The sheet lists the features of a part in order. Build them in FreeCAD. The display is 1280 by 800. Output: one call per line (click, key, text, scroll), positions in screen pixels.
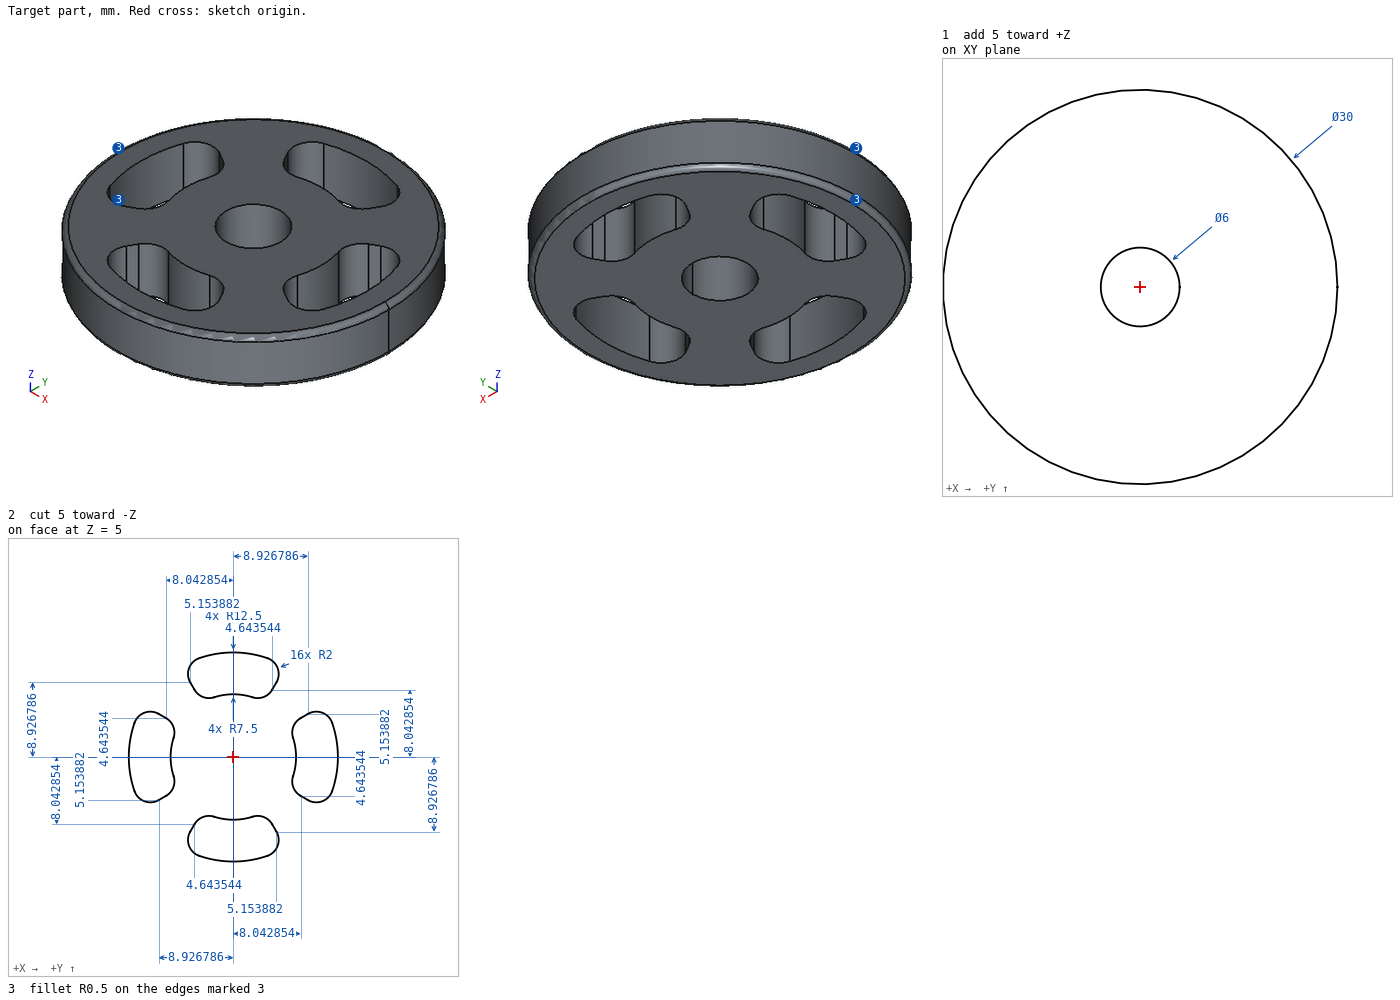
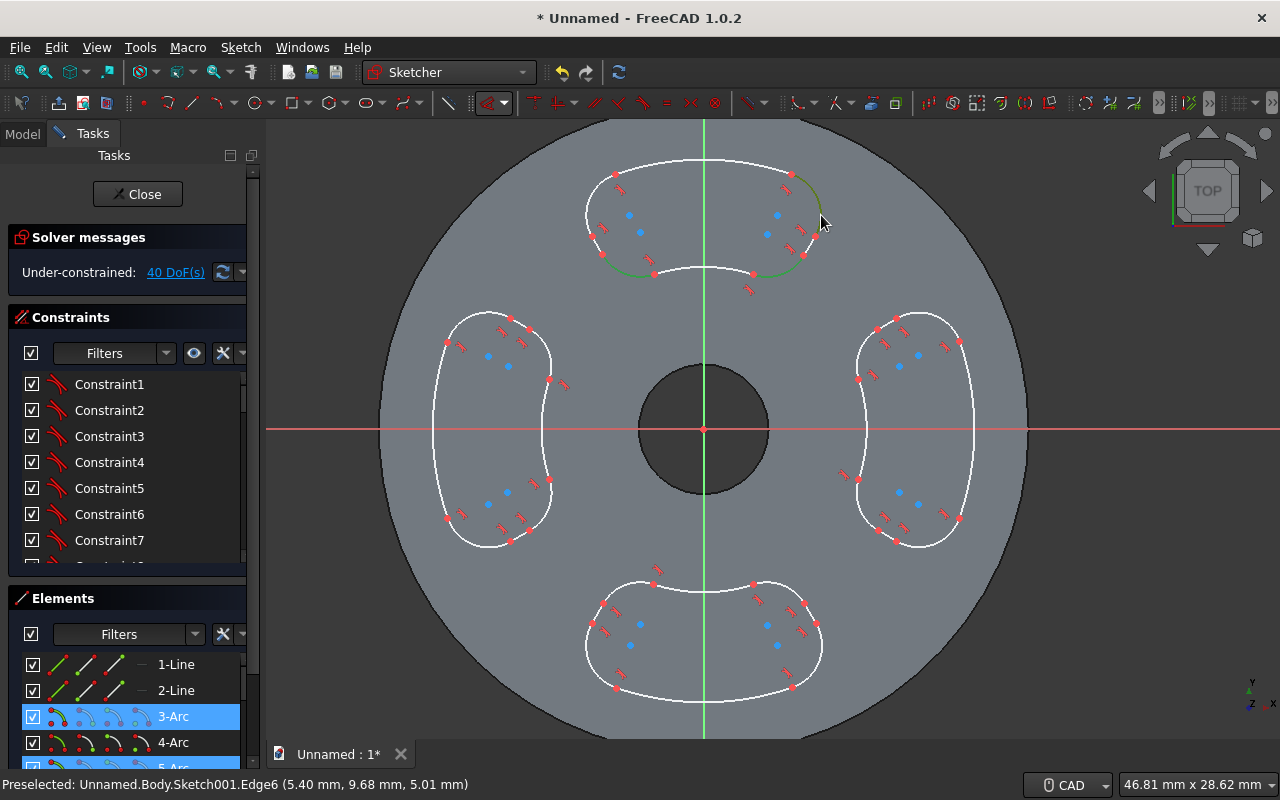
click(597, 187)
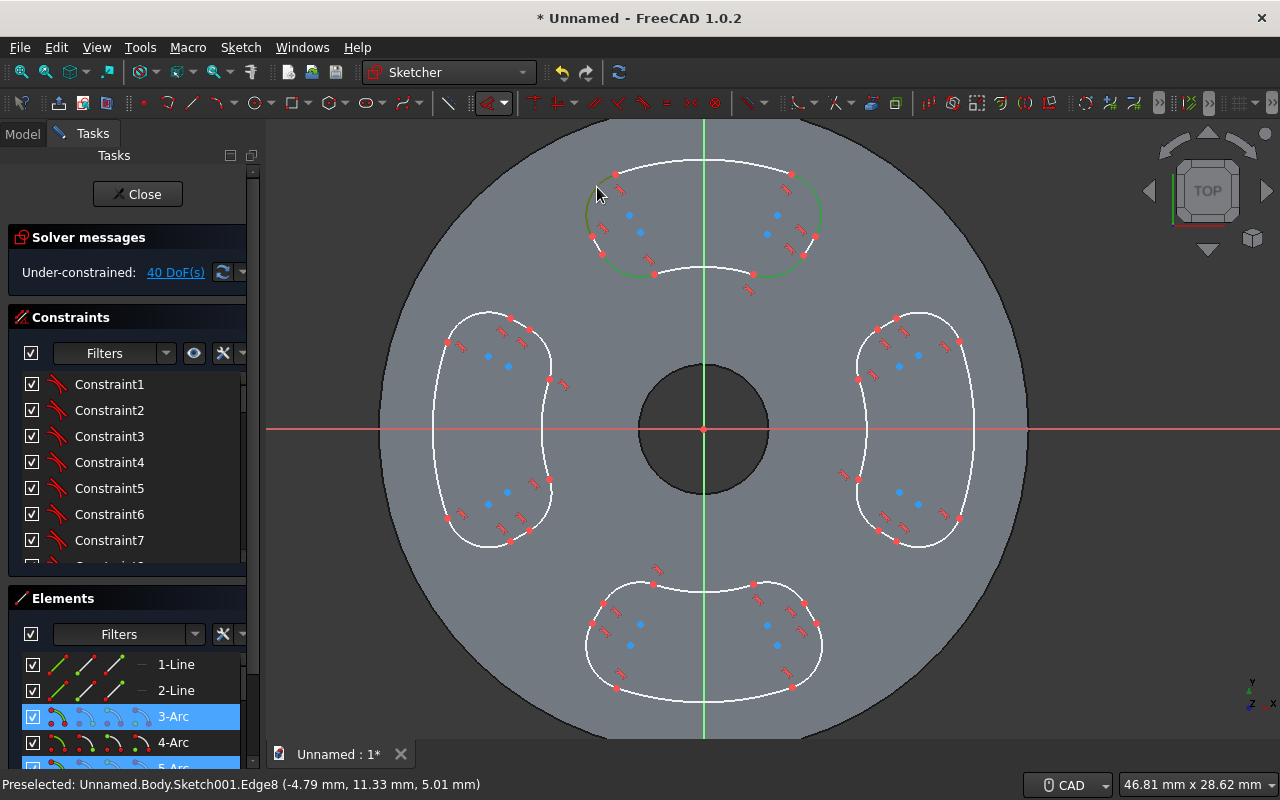
click(865, 341)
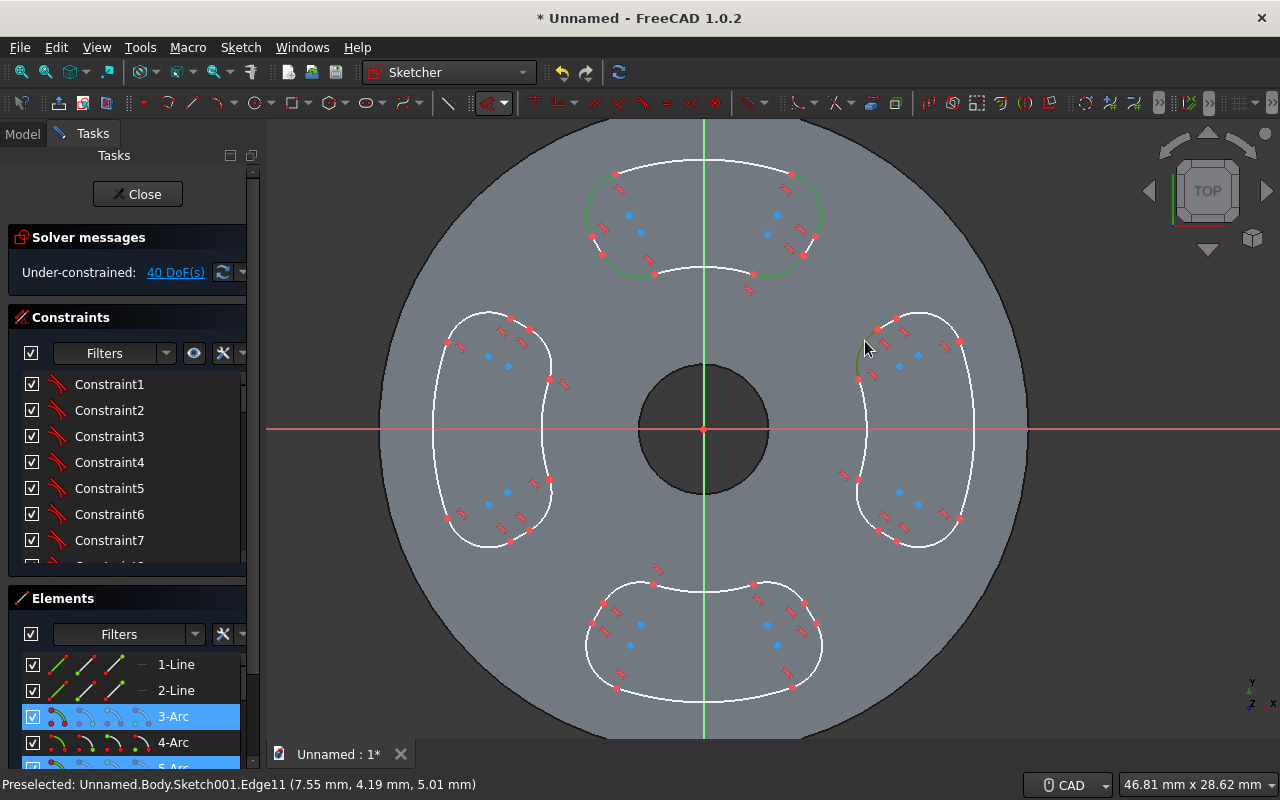
click(857, 497)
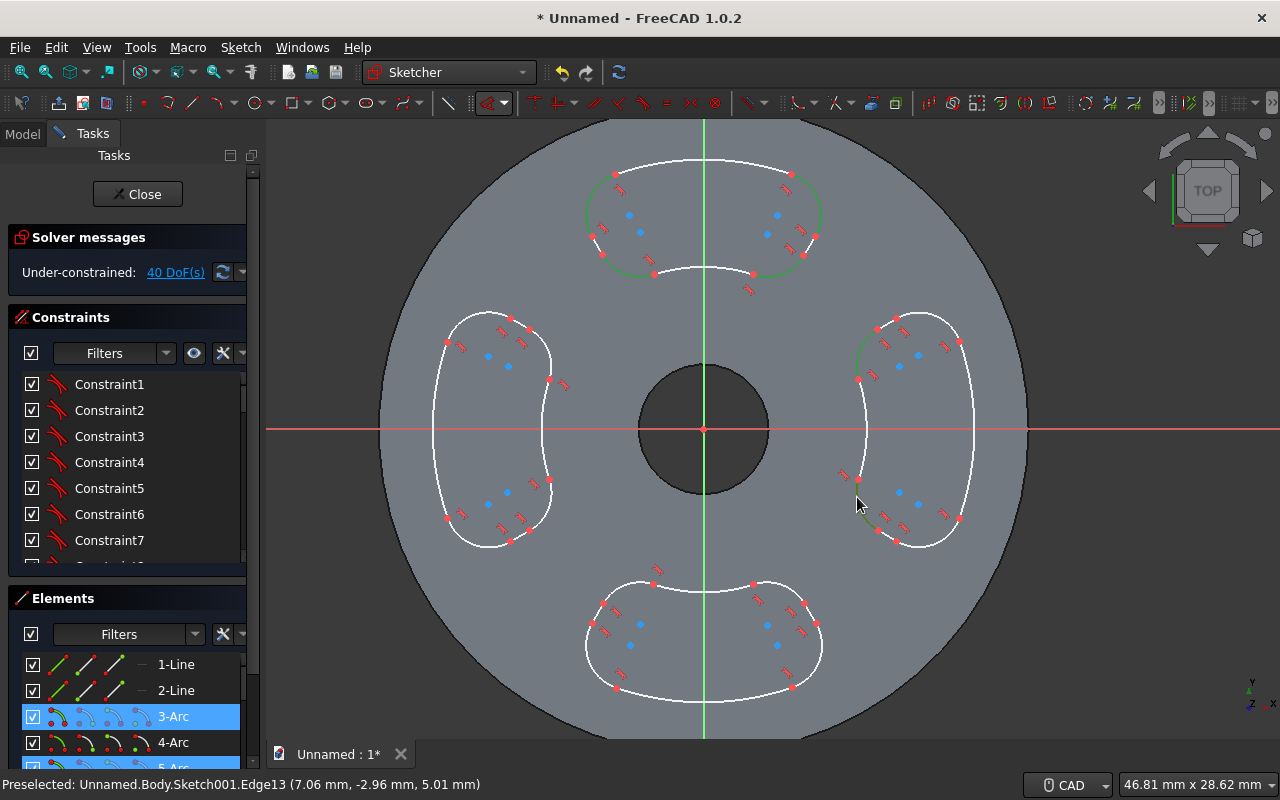
click(919, 547)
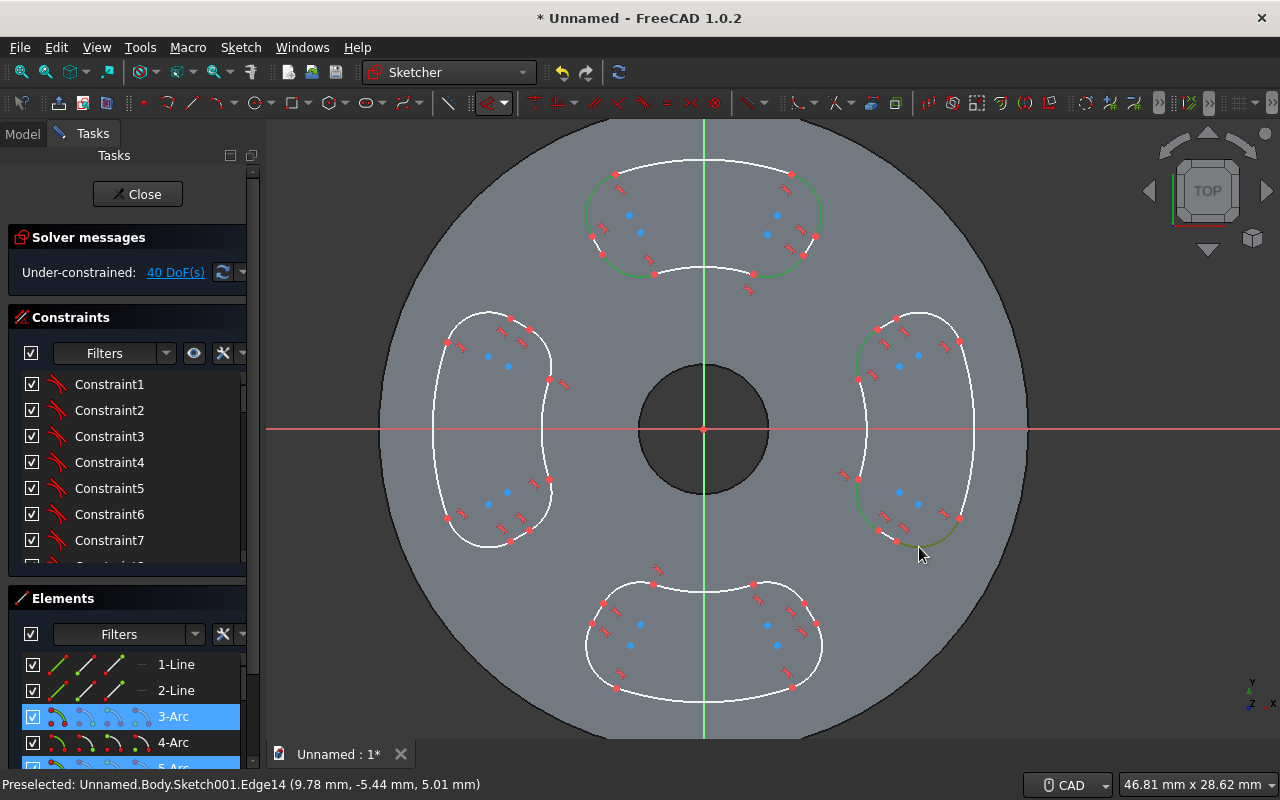
click(947, 323)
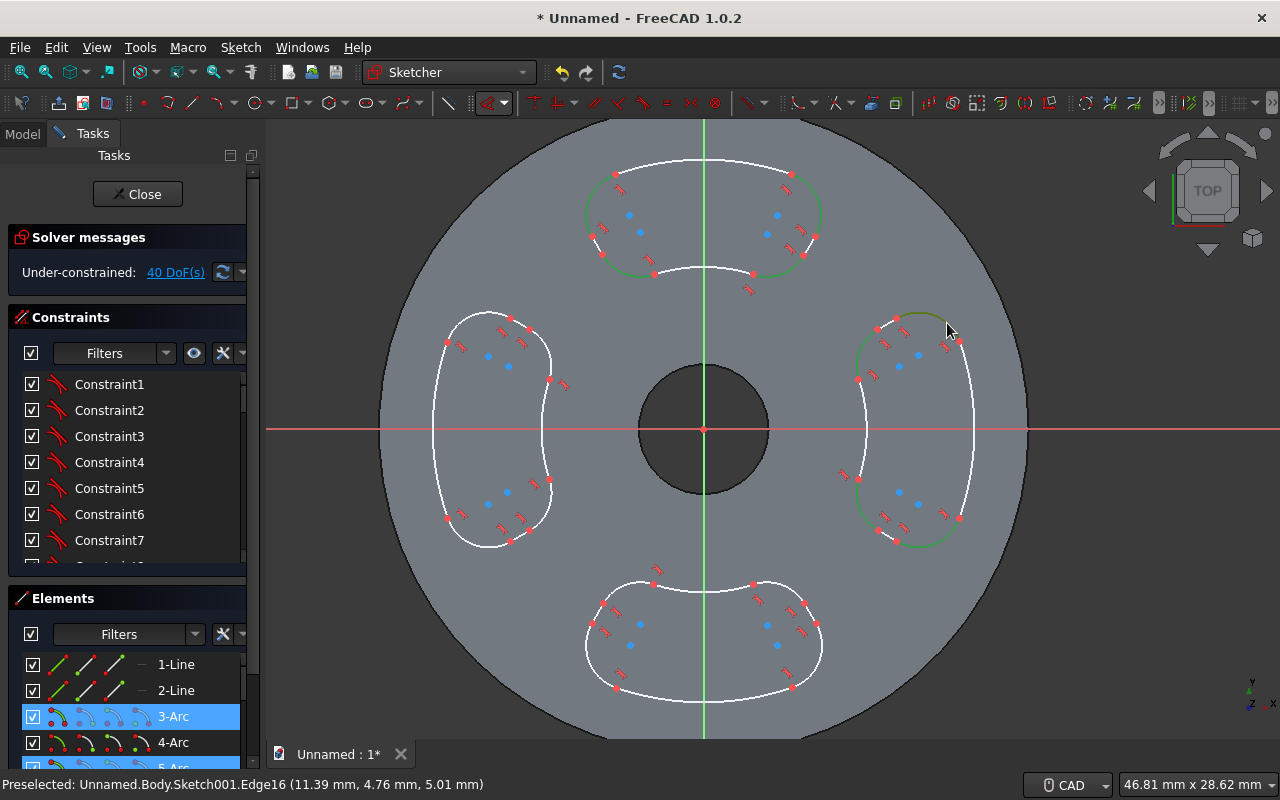
click(793, 591)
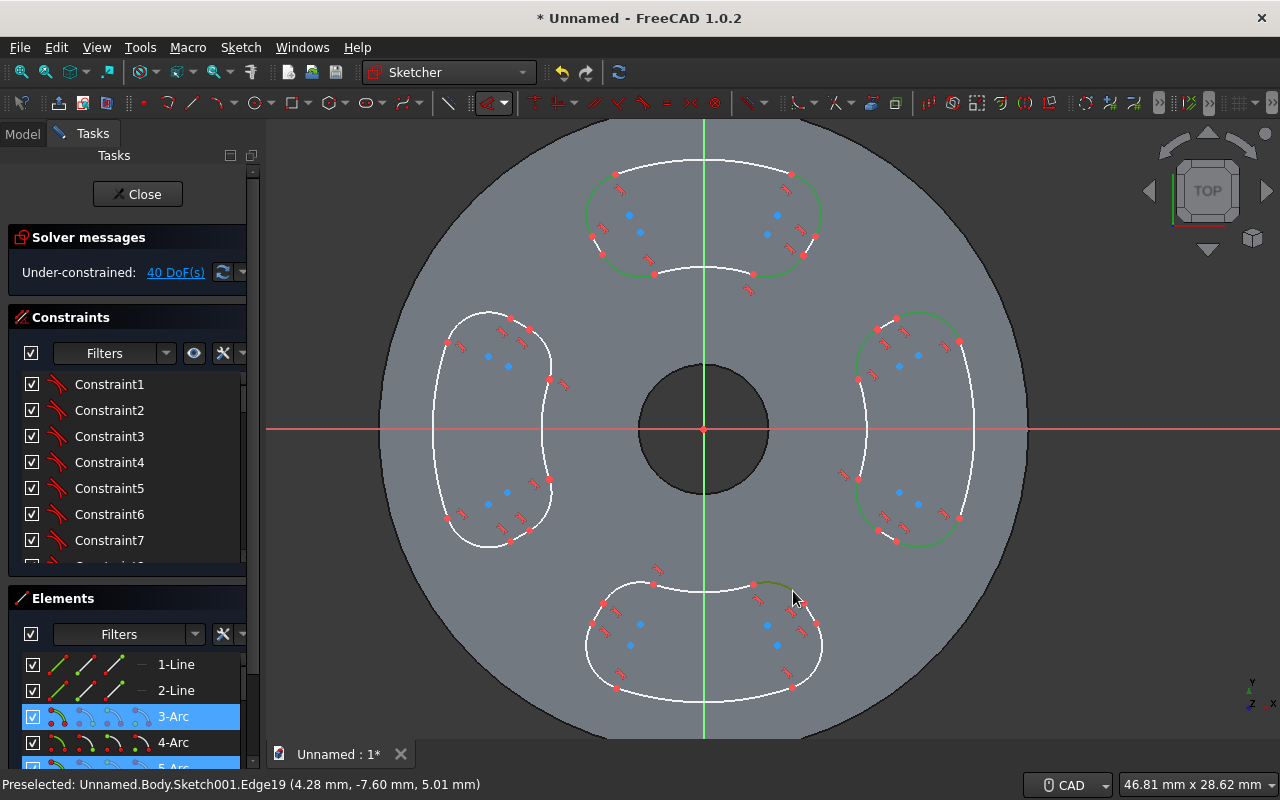
click(636, 582)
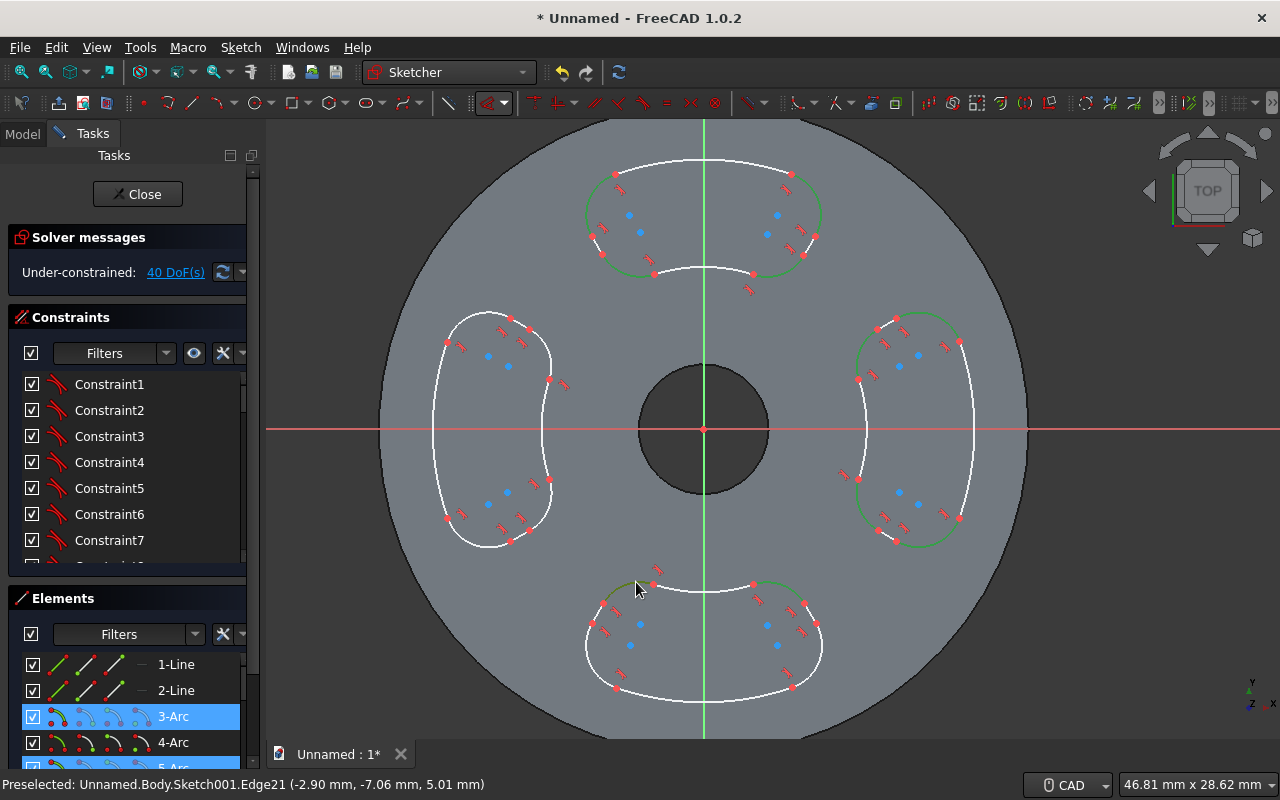
click(586, 646)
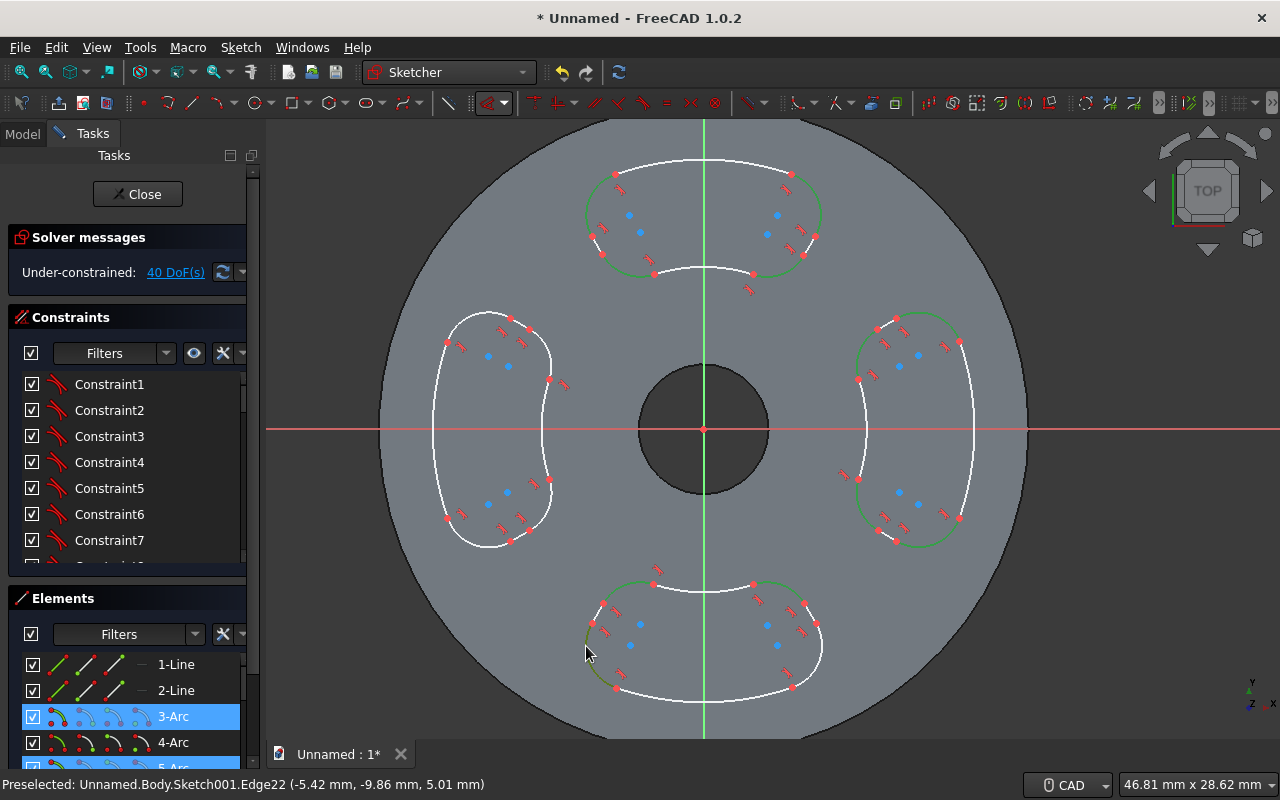
click(811, 675)